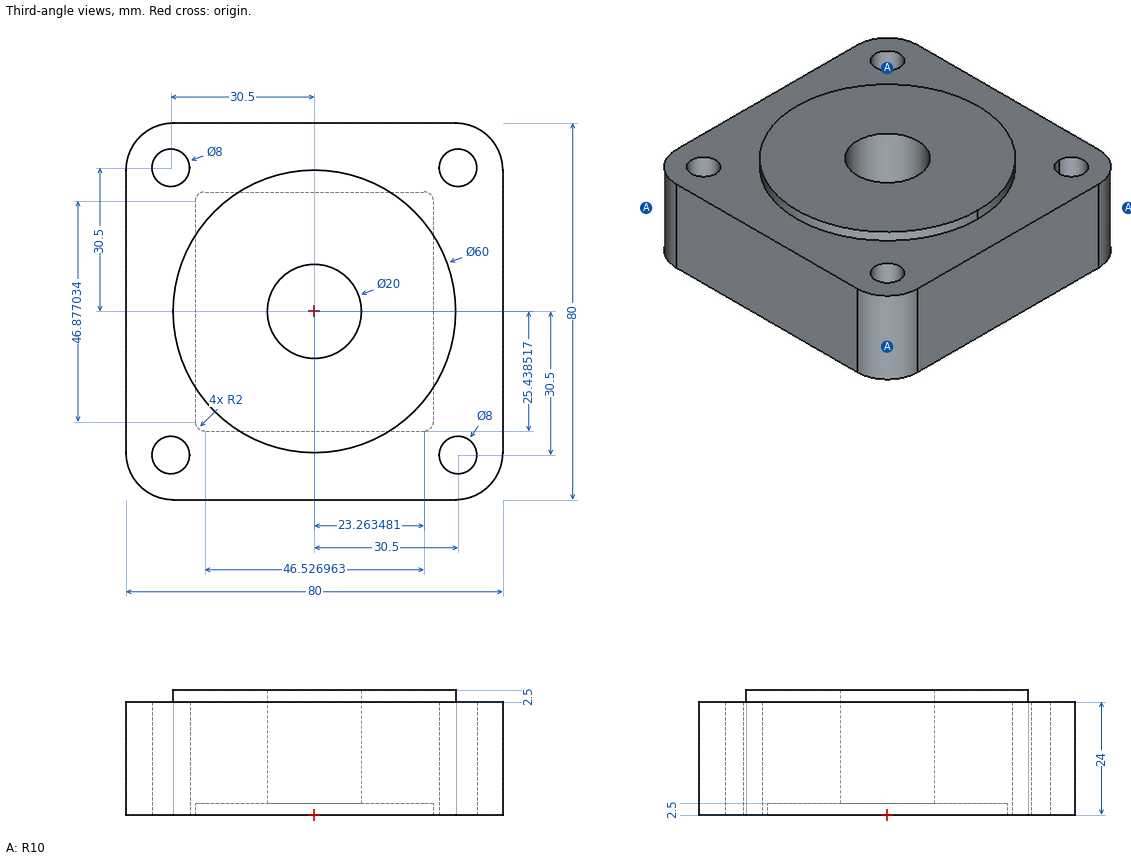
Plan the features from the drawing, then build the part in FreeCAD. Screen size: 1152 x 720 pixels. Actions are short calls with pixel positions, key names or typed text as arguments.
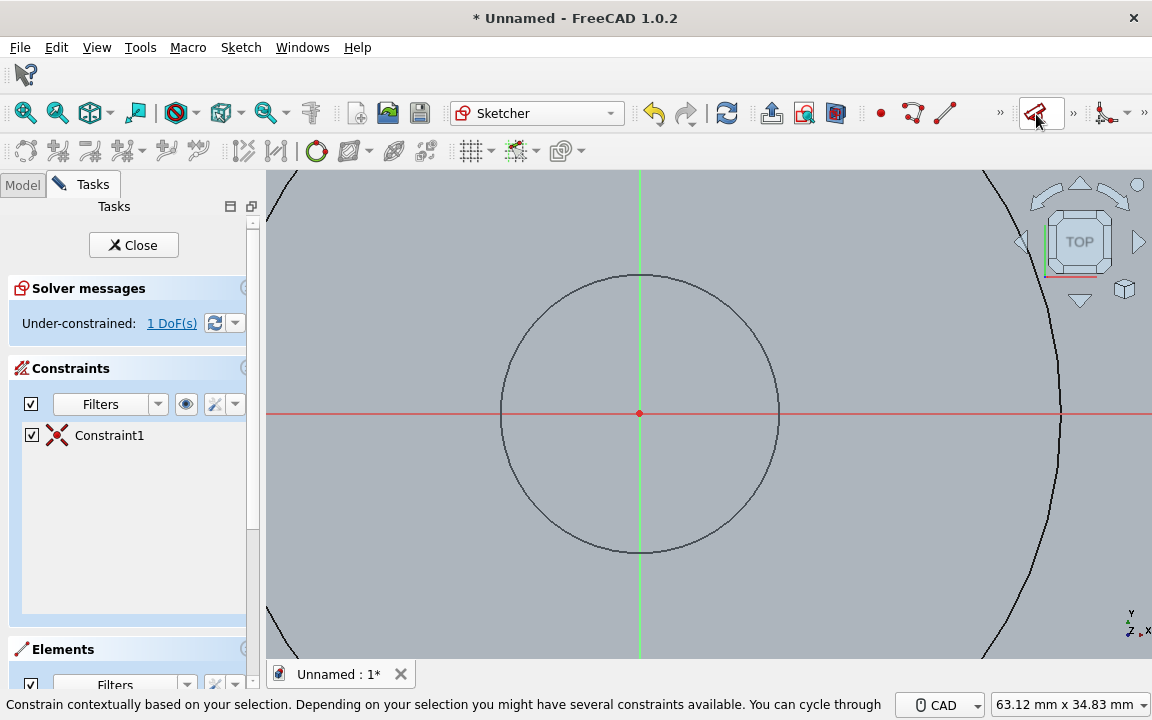
click(738, 315)
click(761, 292)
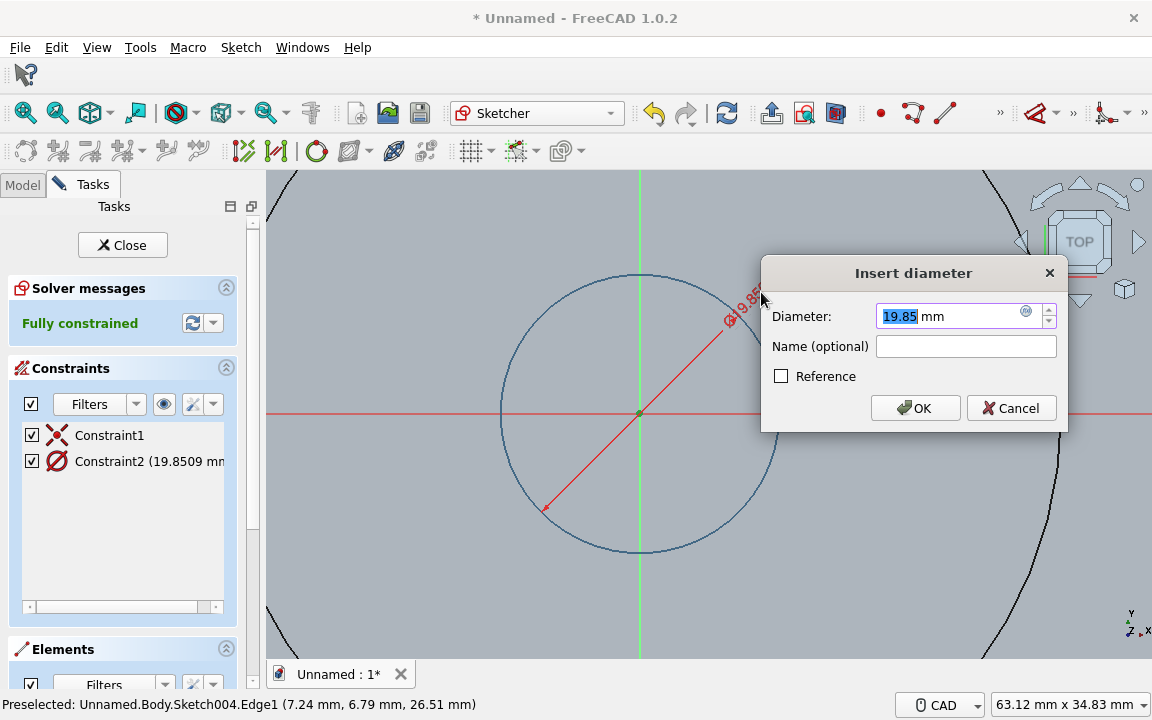
text(20)
key(Return)
key(Escape)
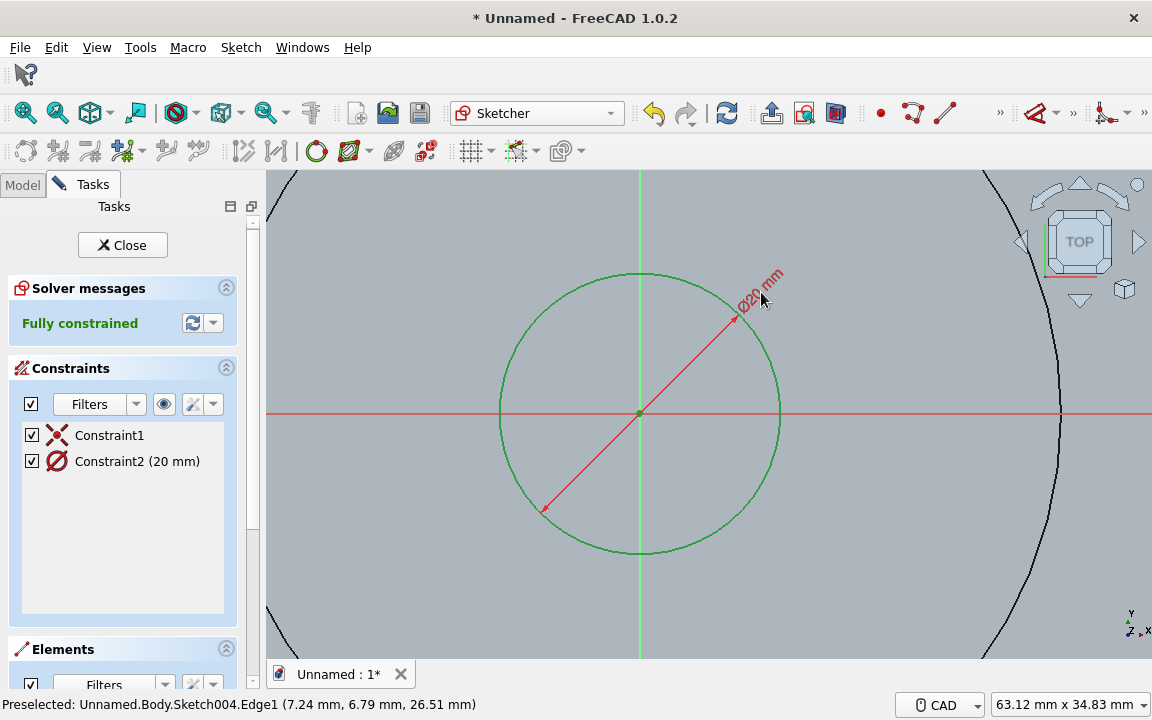
click(123, 245)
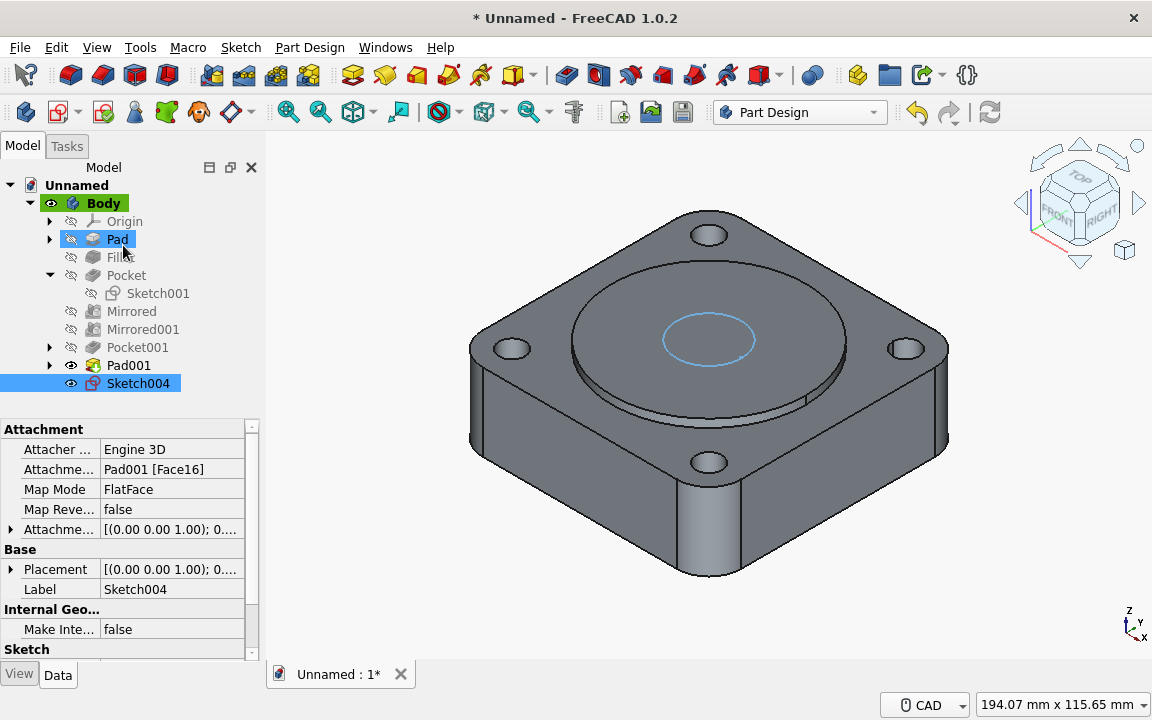
click(568, 76)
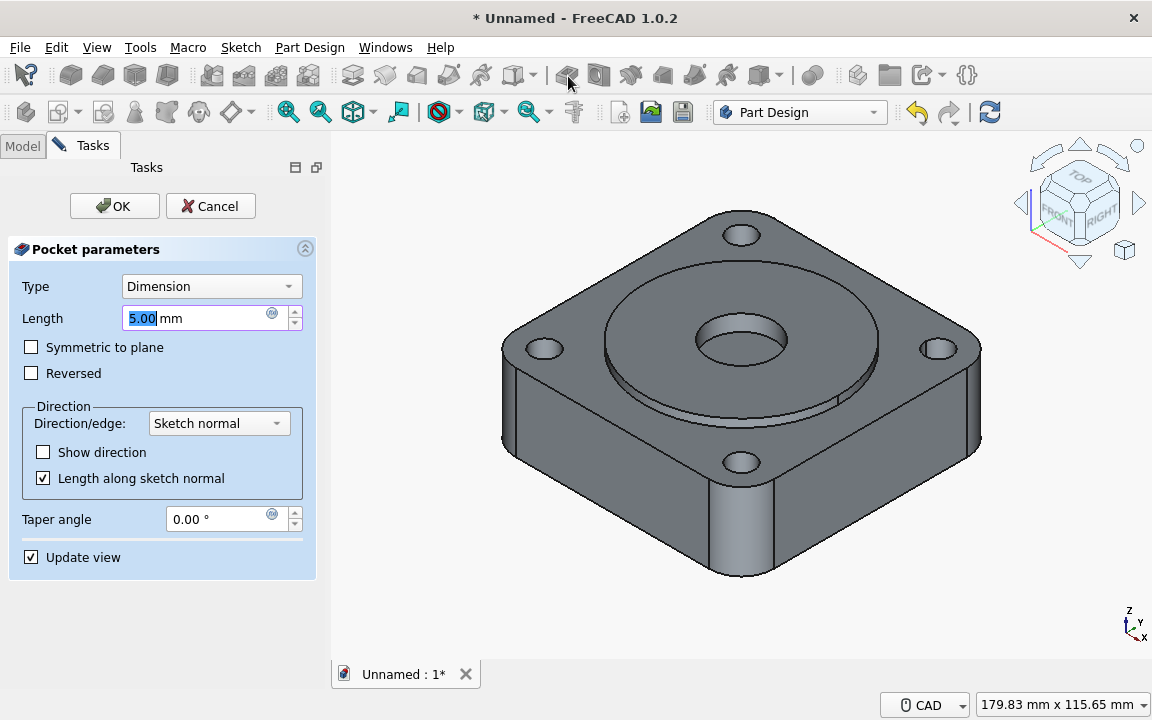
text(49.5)
key(Tab)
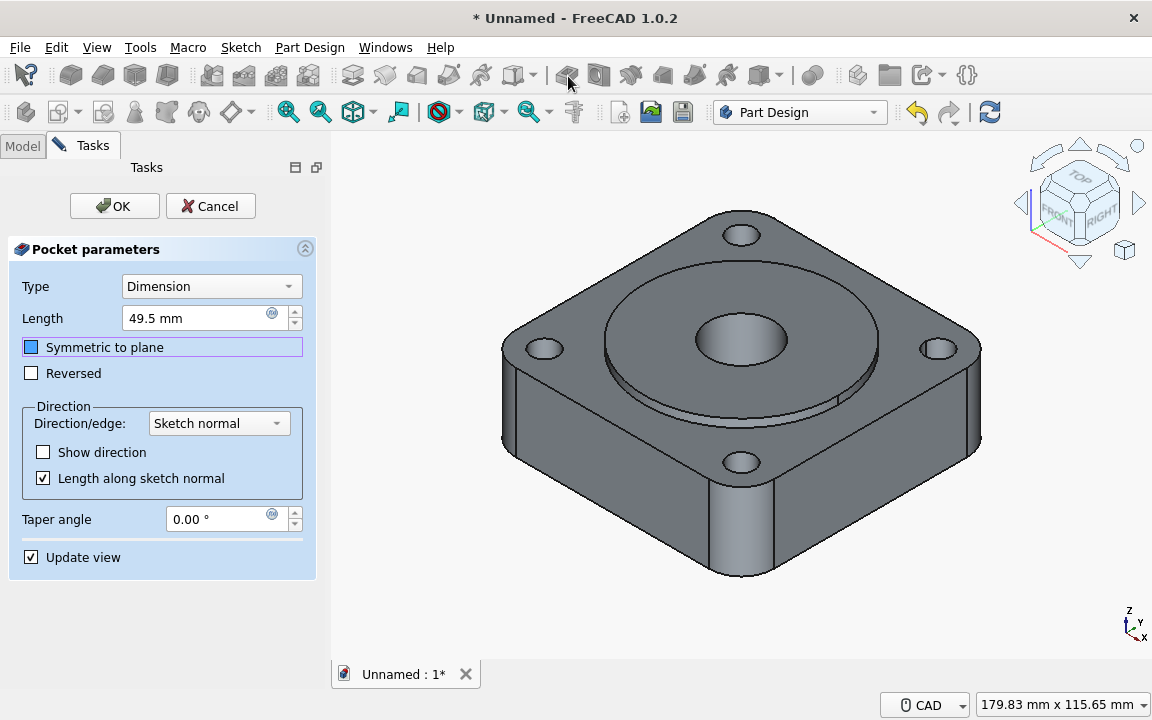
click(115, 206)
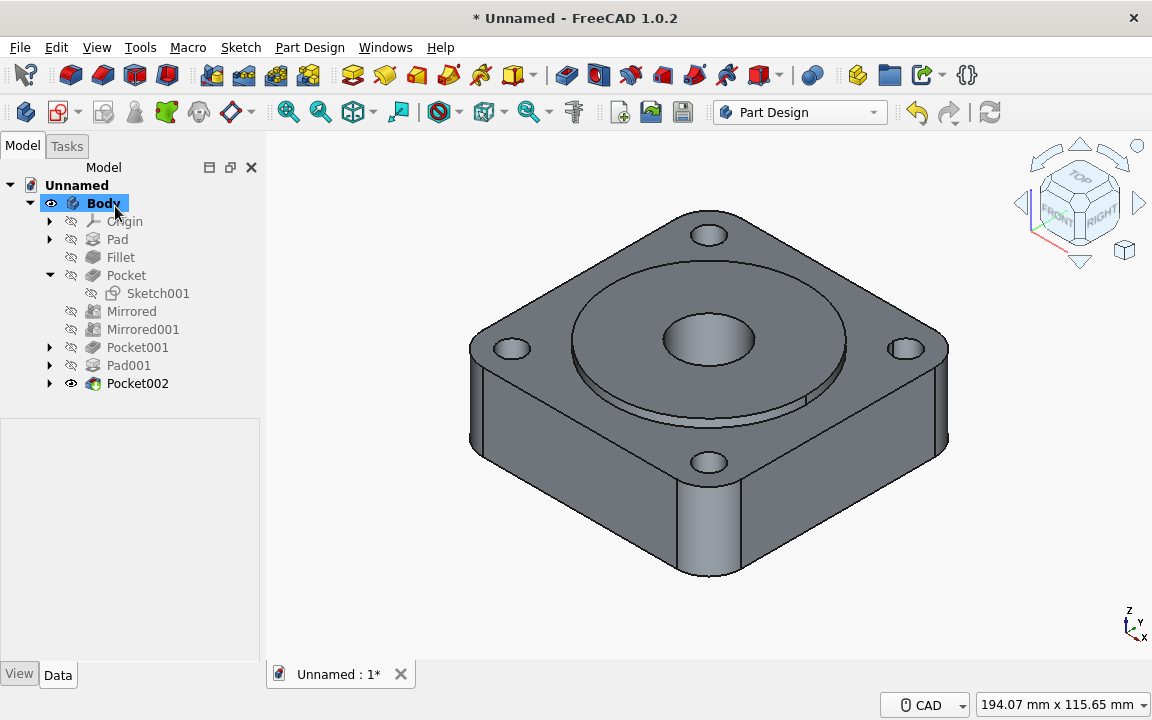
click(58, 112)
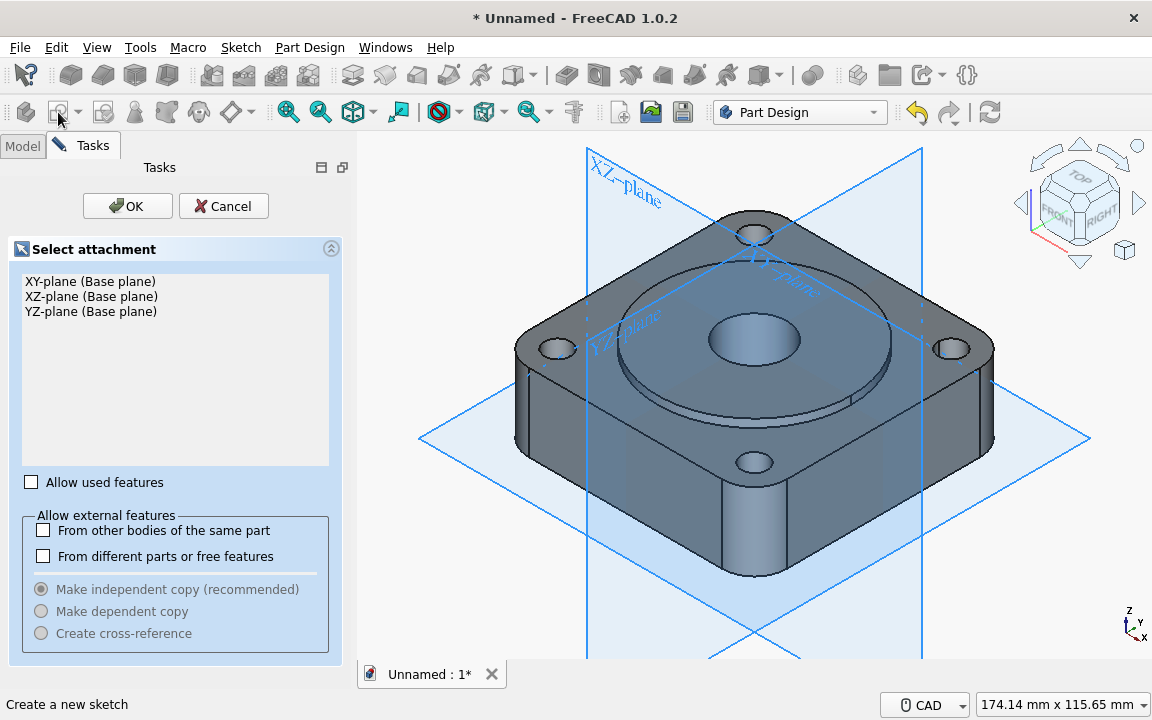
click(82, 282)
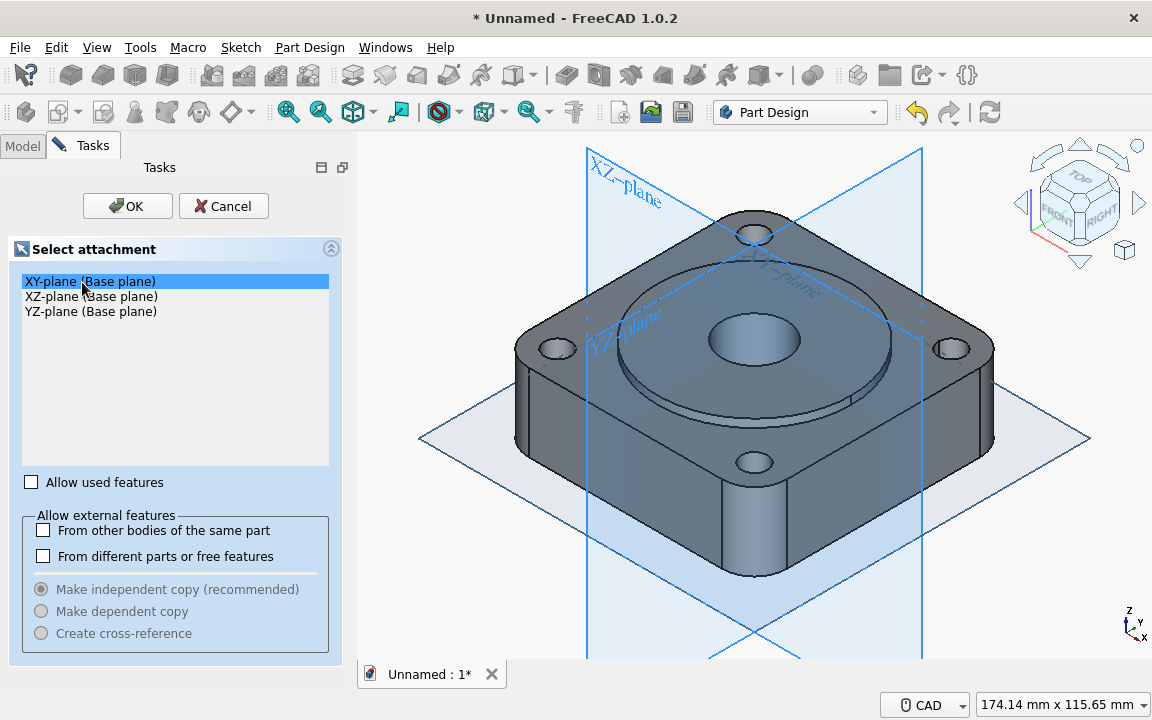
click(128, 206)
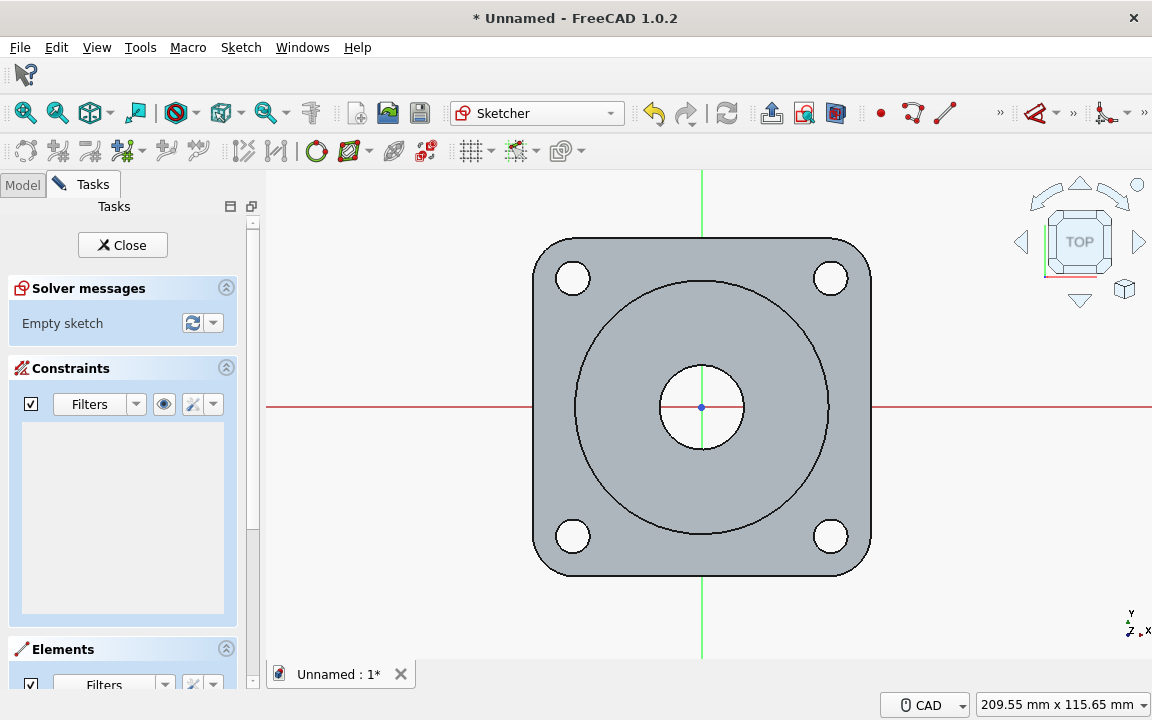
click(836, 114)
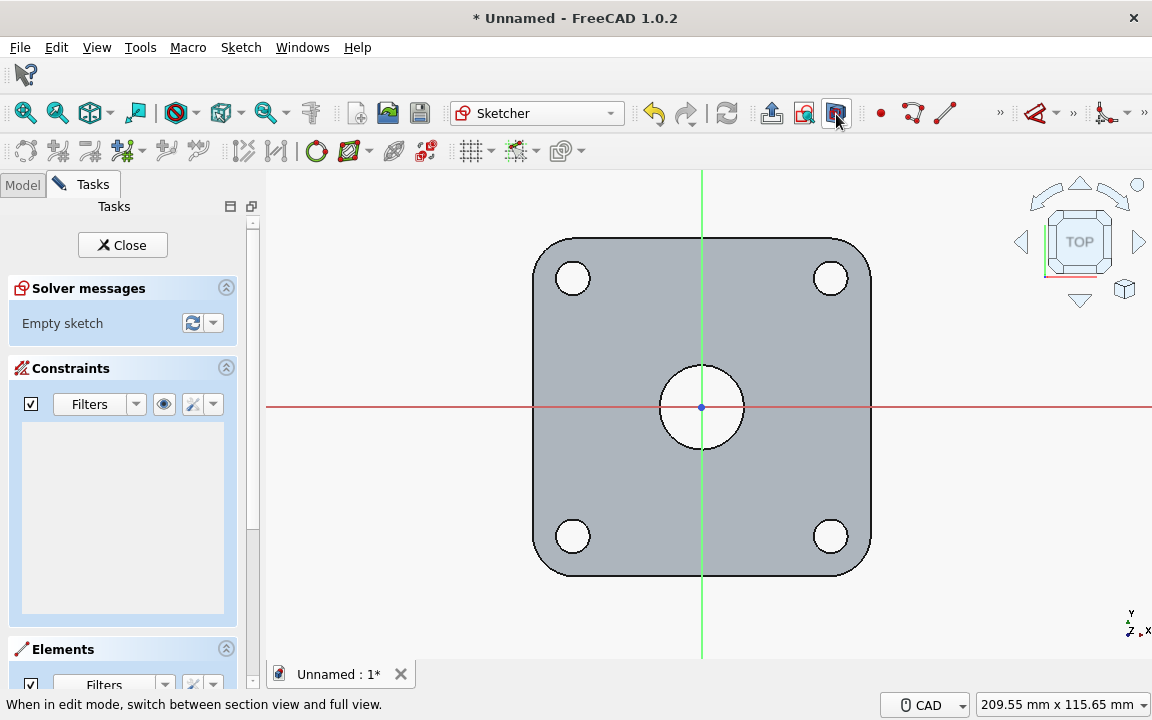
scroll(827, 393, up, 2)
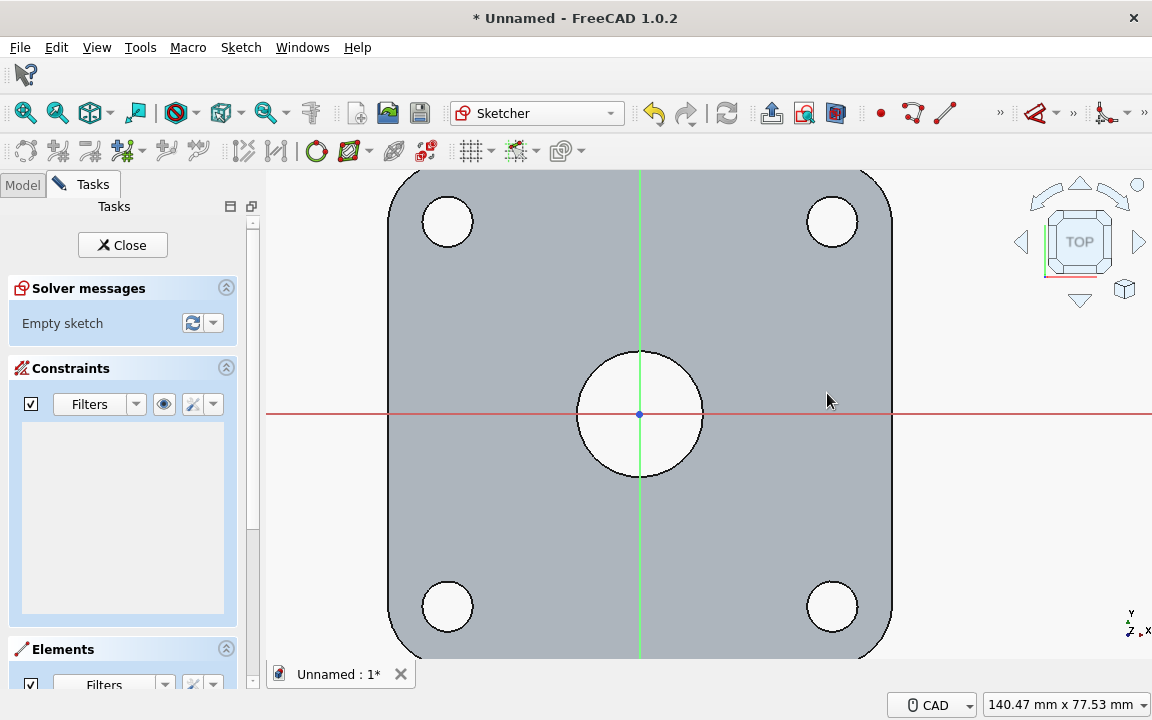
click(946, 114)